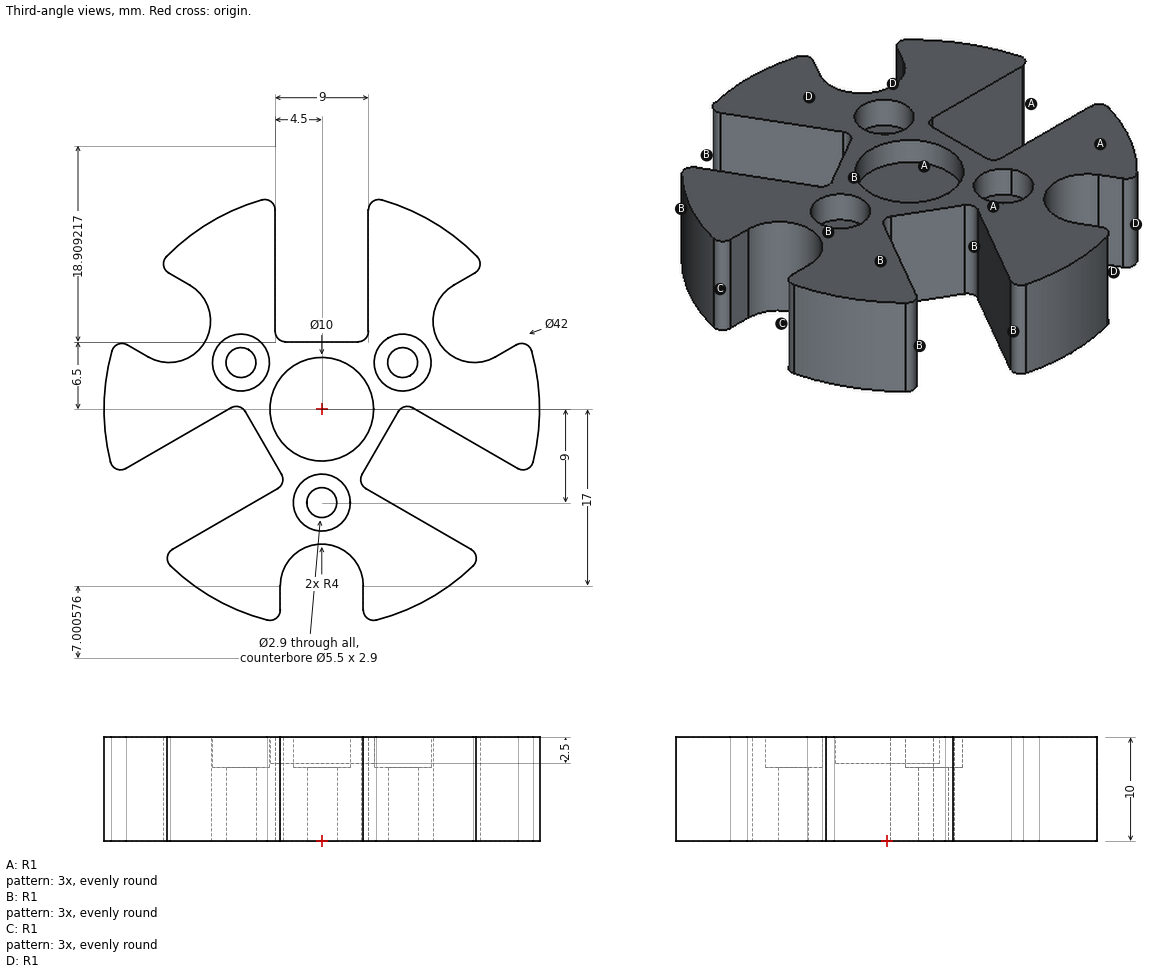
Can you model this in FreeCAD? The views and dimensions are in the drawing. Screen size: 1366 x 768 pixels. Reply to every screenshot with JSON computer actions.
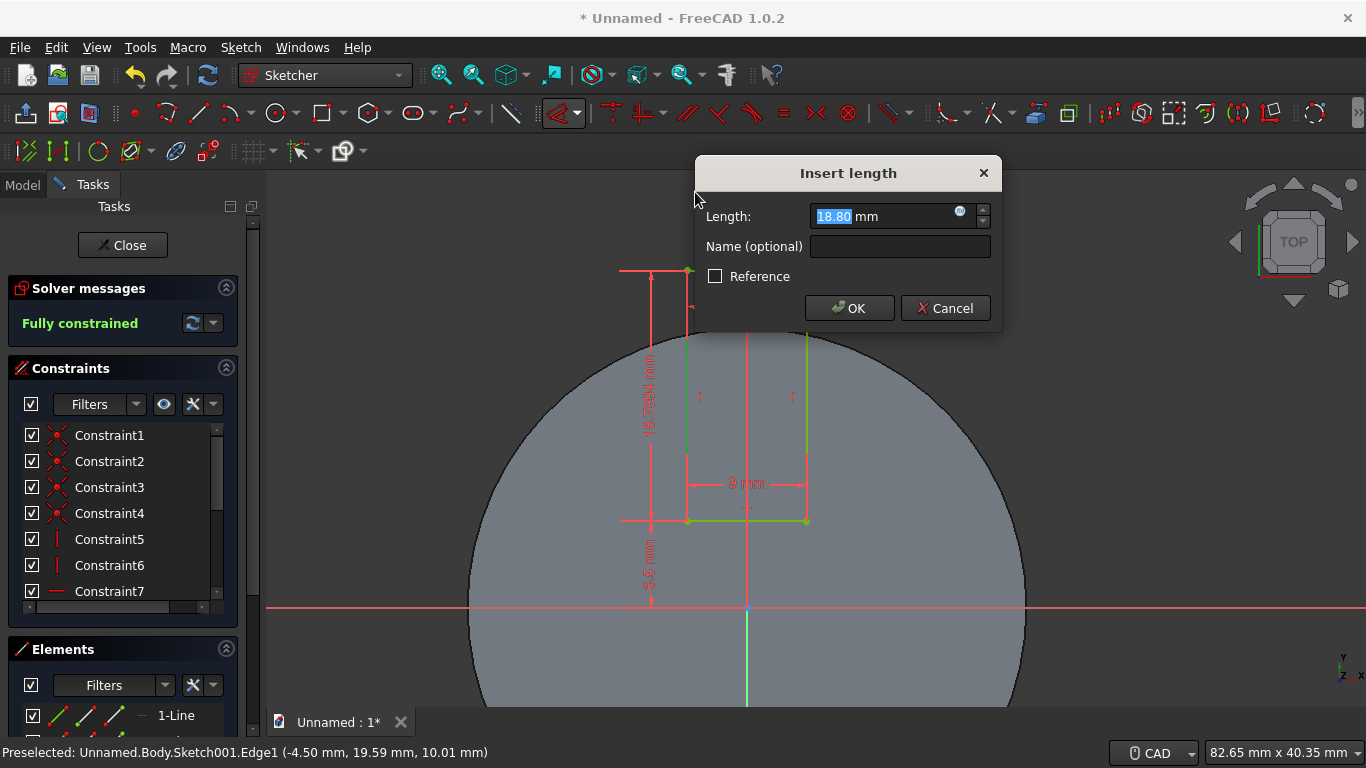
{"action": "type", "text": "18.909217"}
{"action": "key", "text": "Return"}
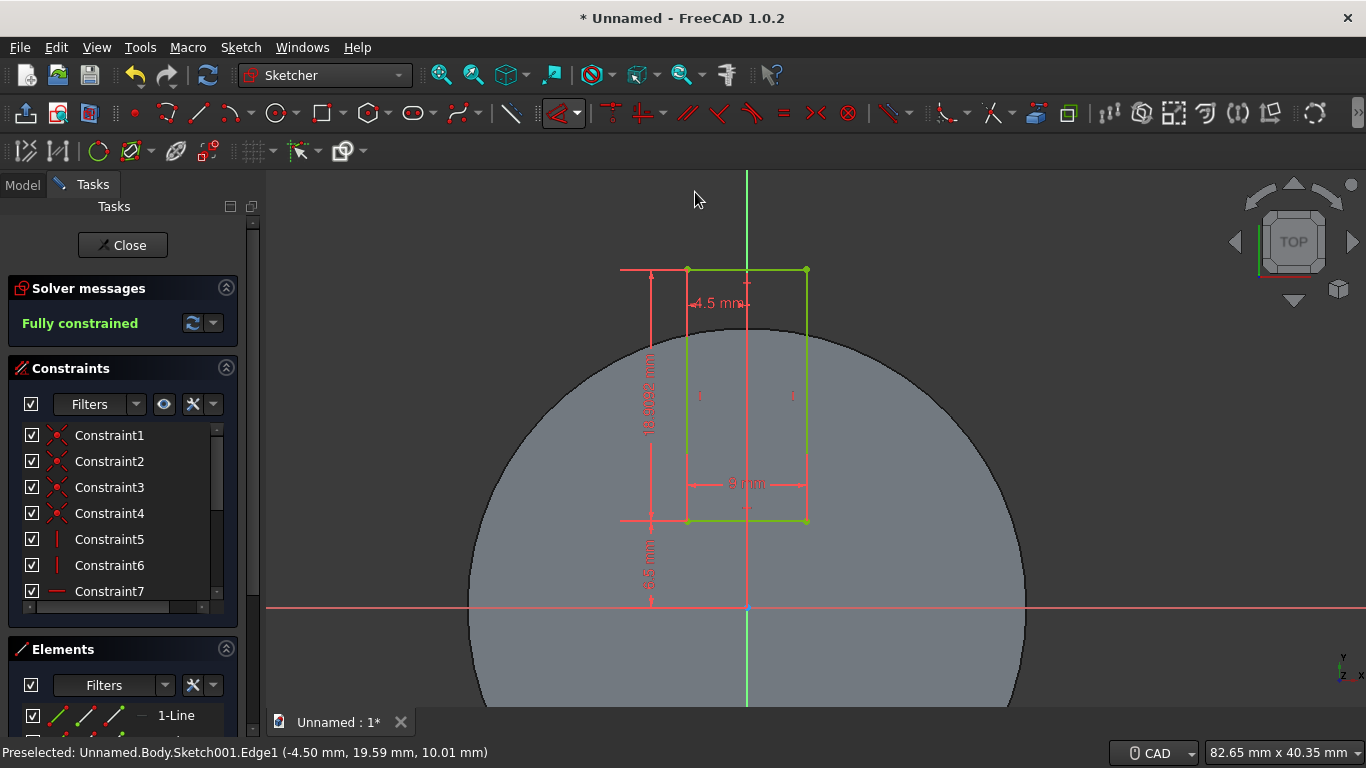
{"action": "left_click", "coordinate": [123, 245]}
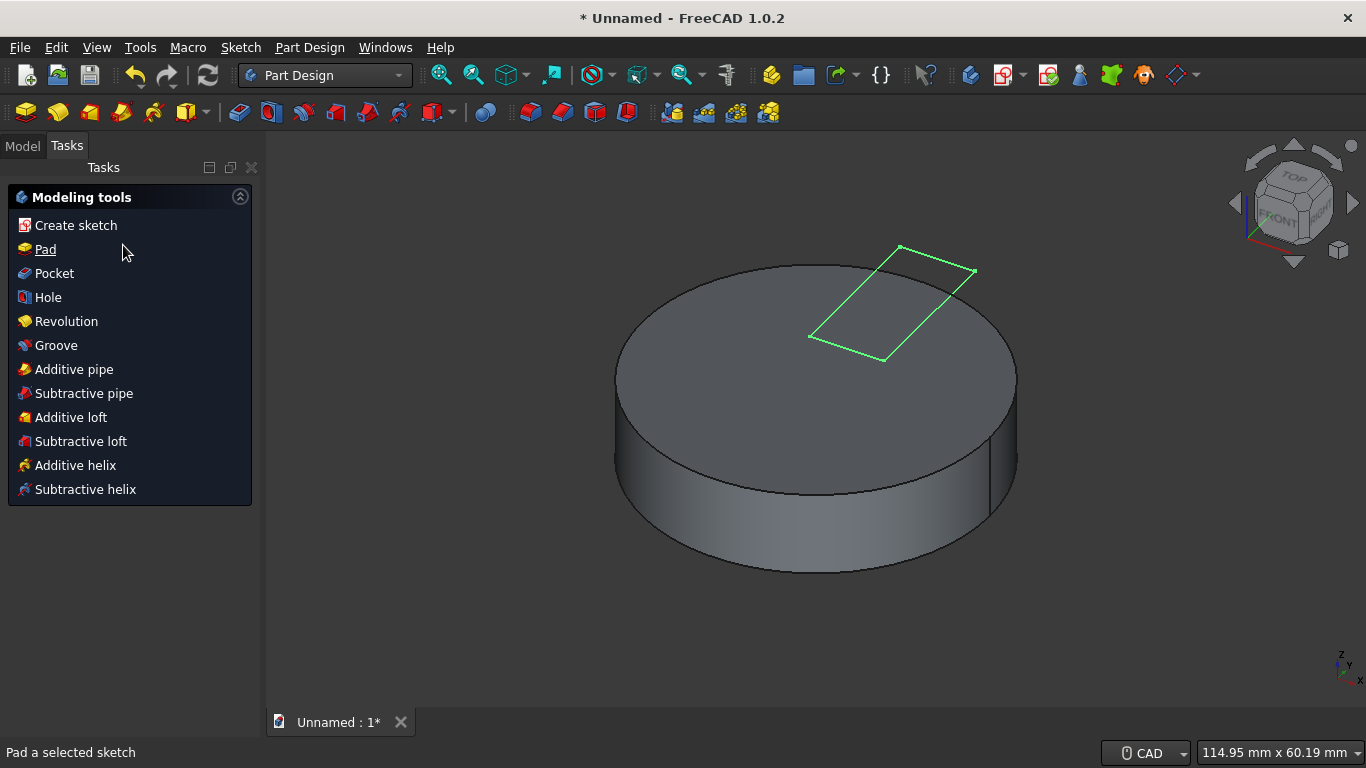
{"action": "left_click", "coordinate": [240, 112]}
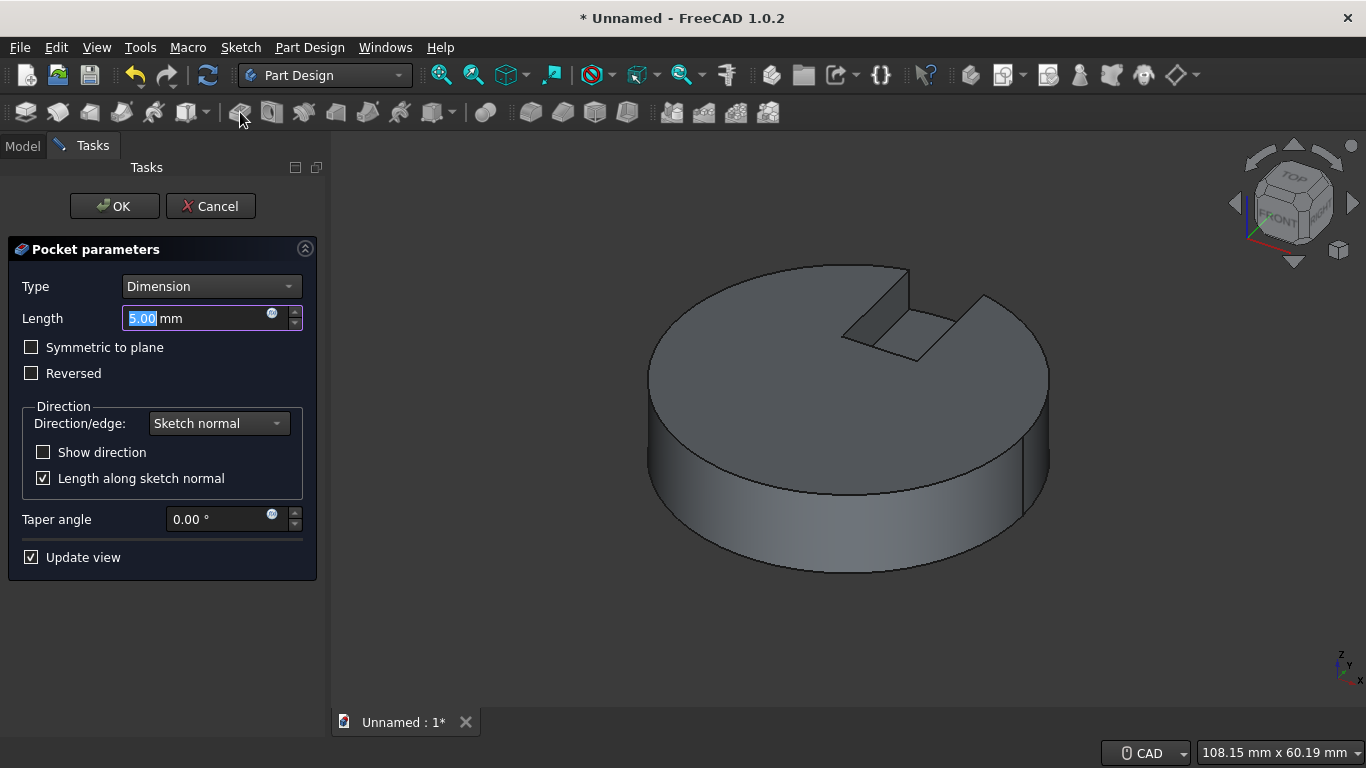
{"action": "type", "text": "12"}
{"action": "key", "text": "Tab"}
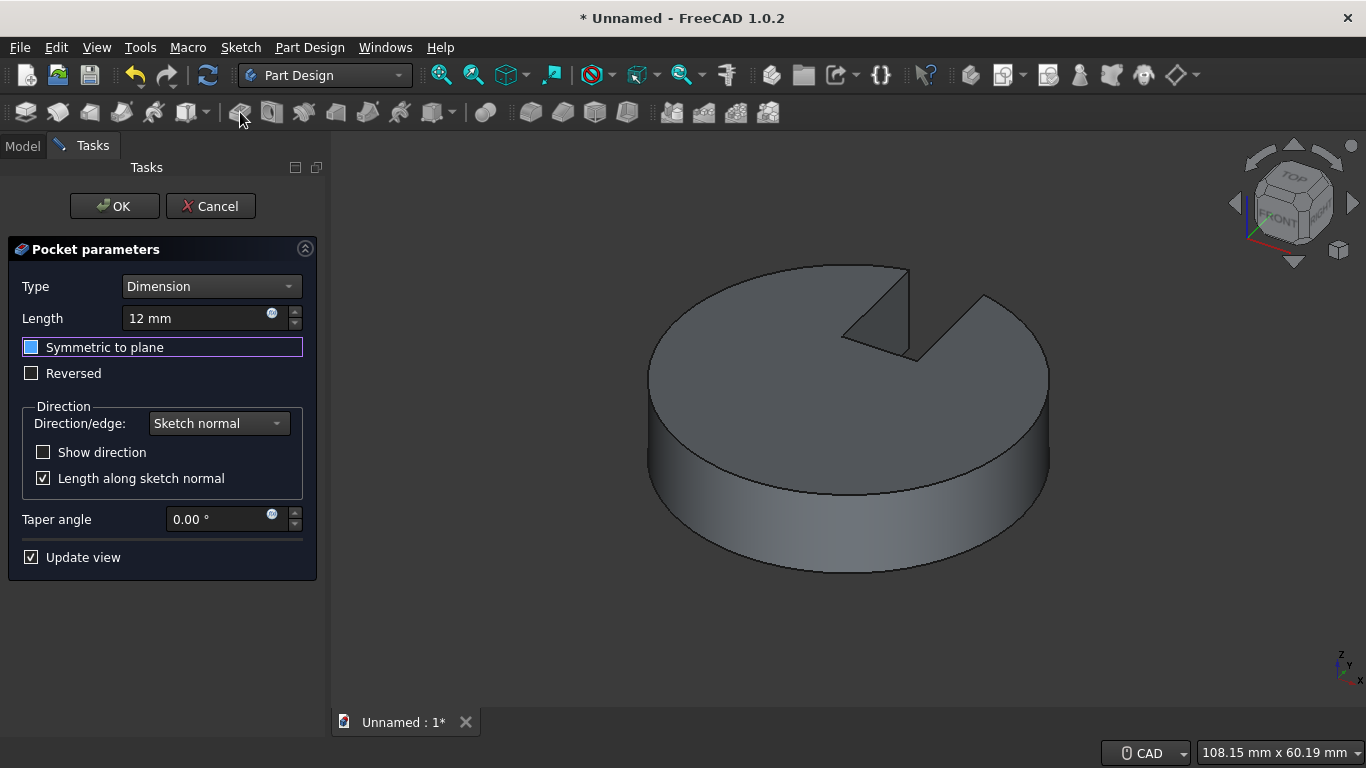
{"action": "left_click", "coordinate": [115, 206]}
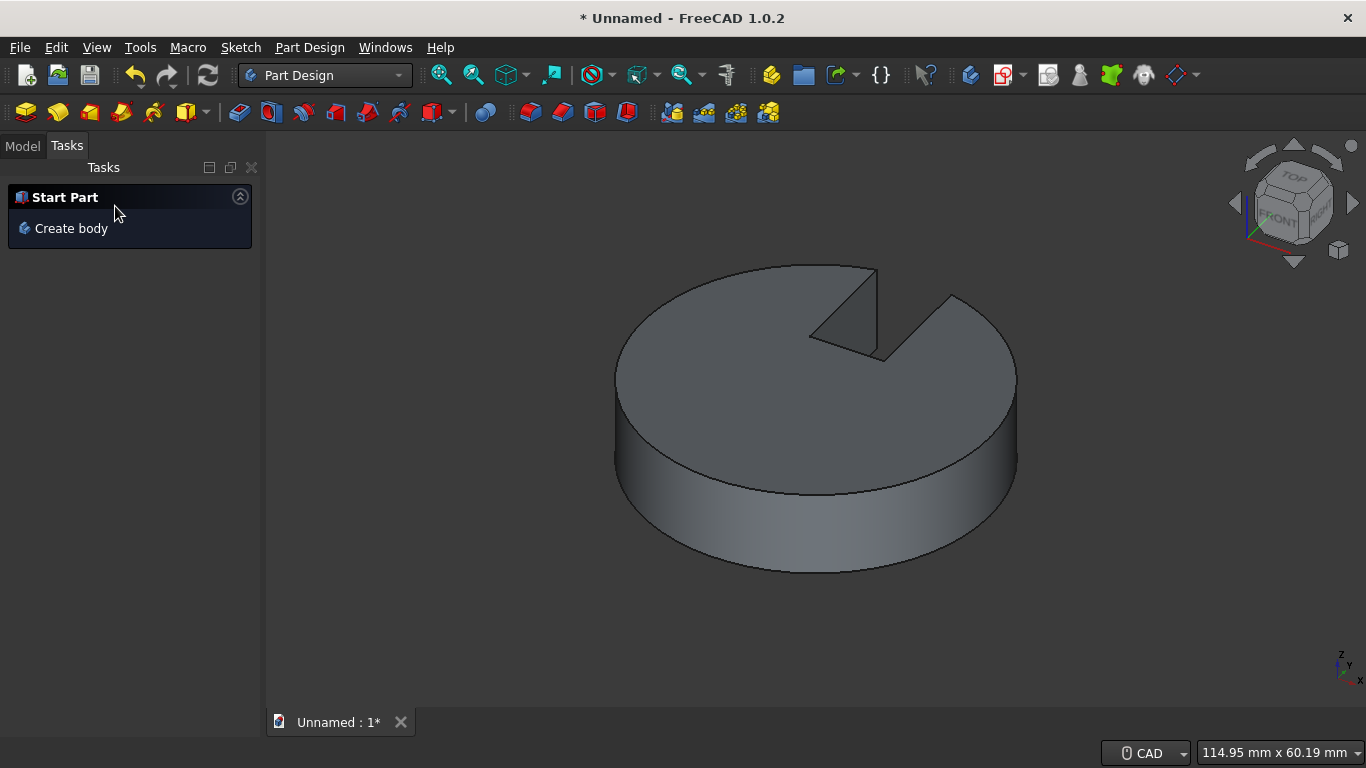
{"action": "key", "text": "0"}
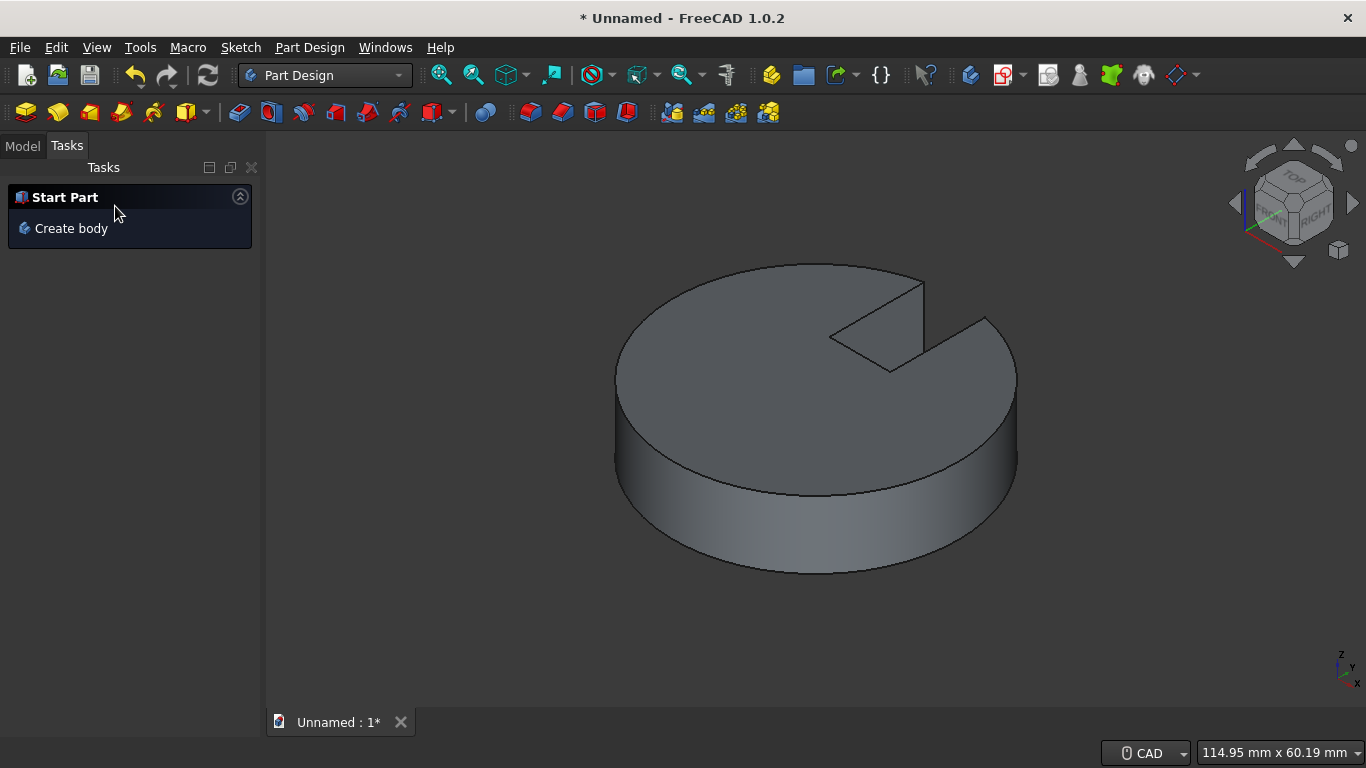
{"action": "key", "text": "2"}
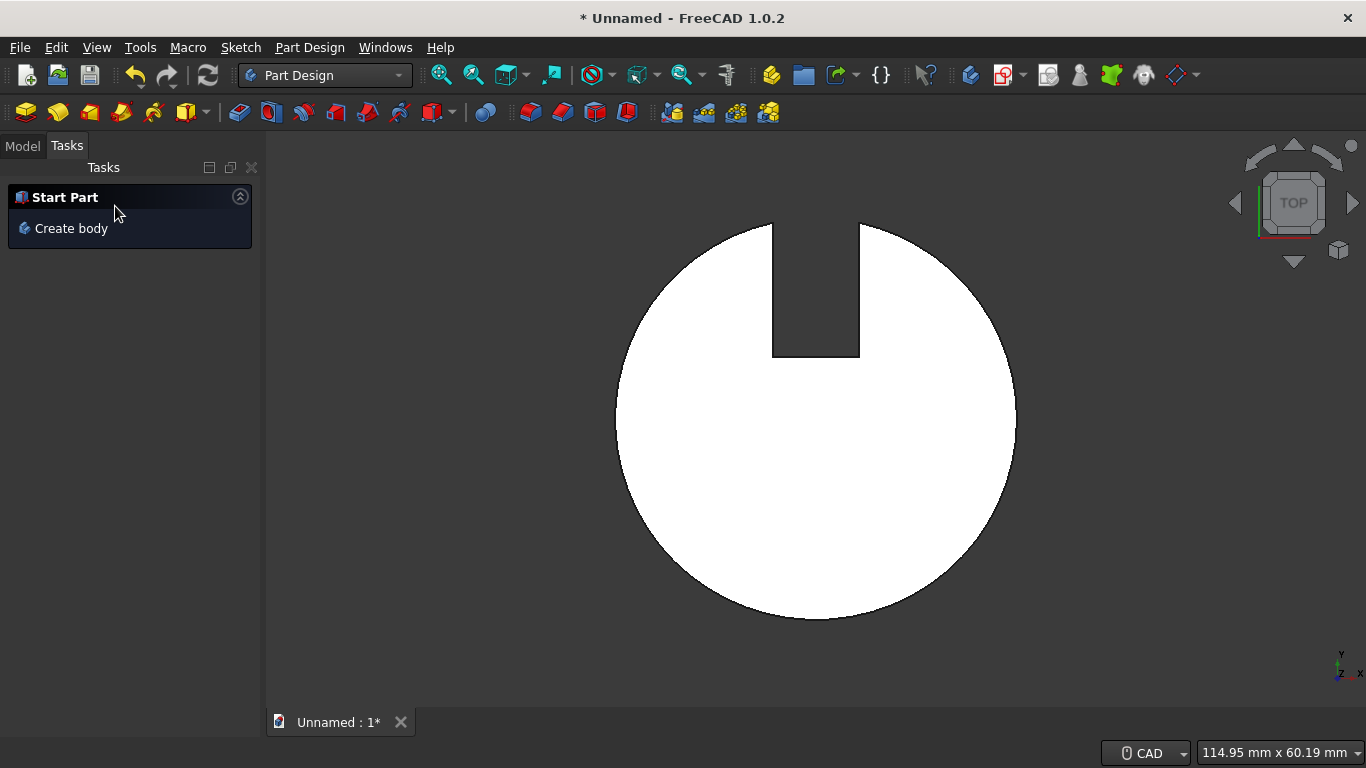
{"action": "key", "text": "1"}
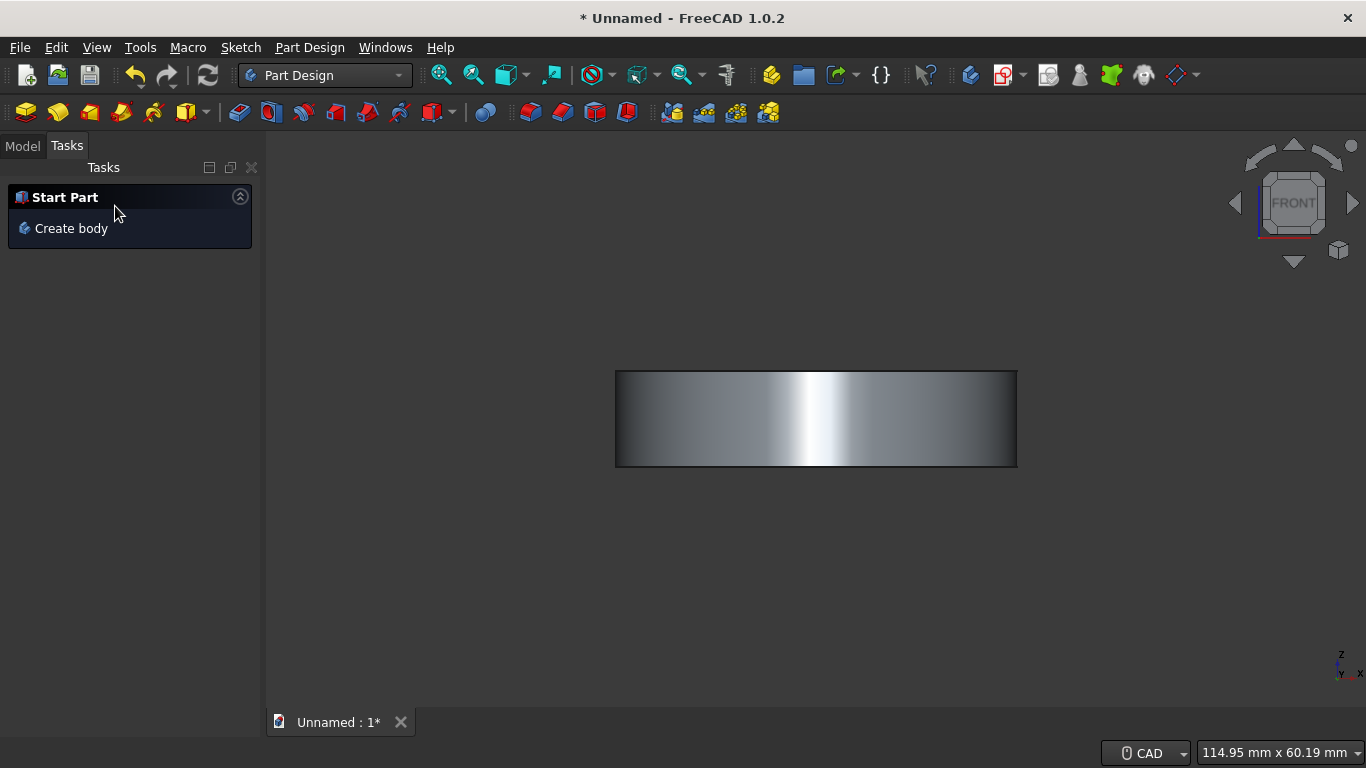
{"action": "left_click", "coordinate": [442, 76]}